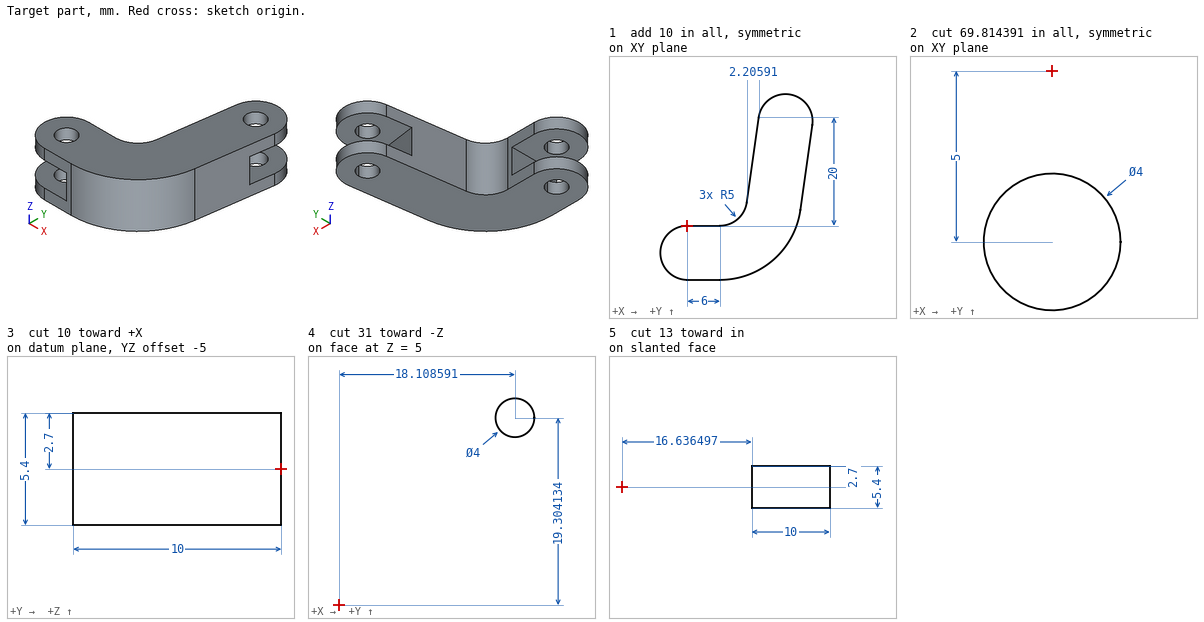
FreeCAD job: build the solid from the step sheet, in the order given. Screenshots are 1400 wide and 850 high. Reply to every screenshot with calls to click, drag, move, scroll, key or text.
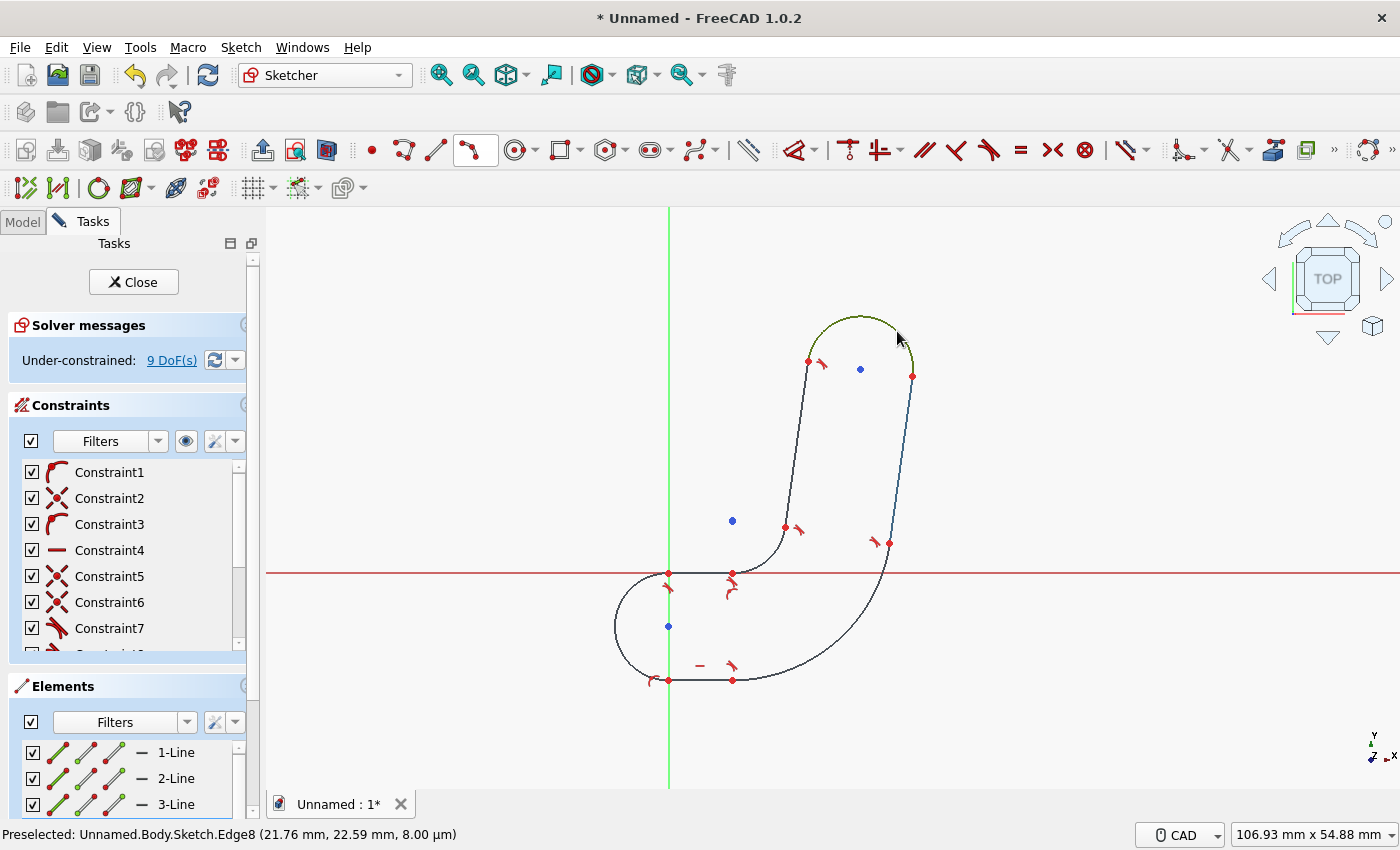
click(990, 150)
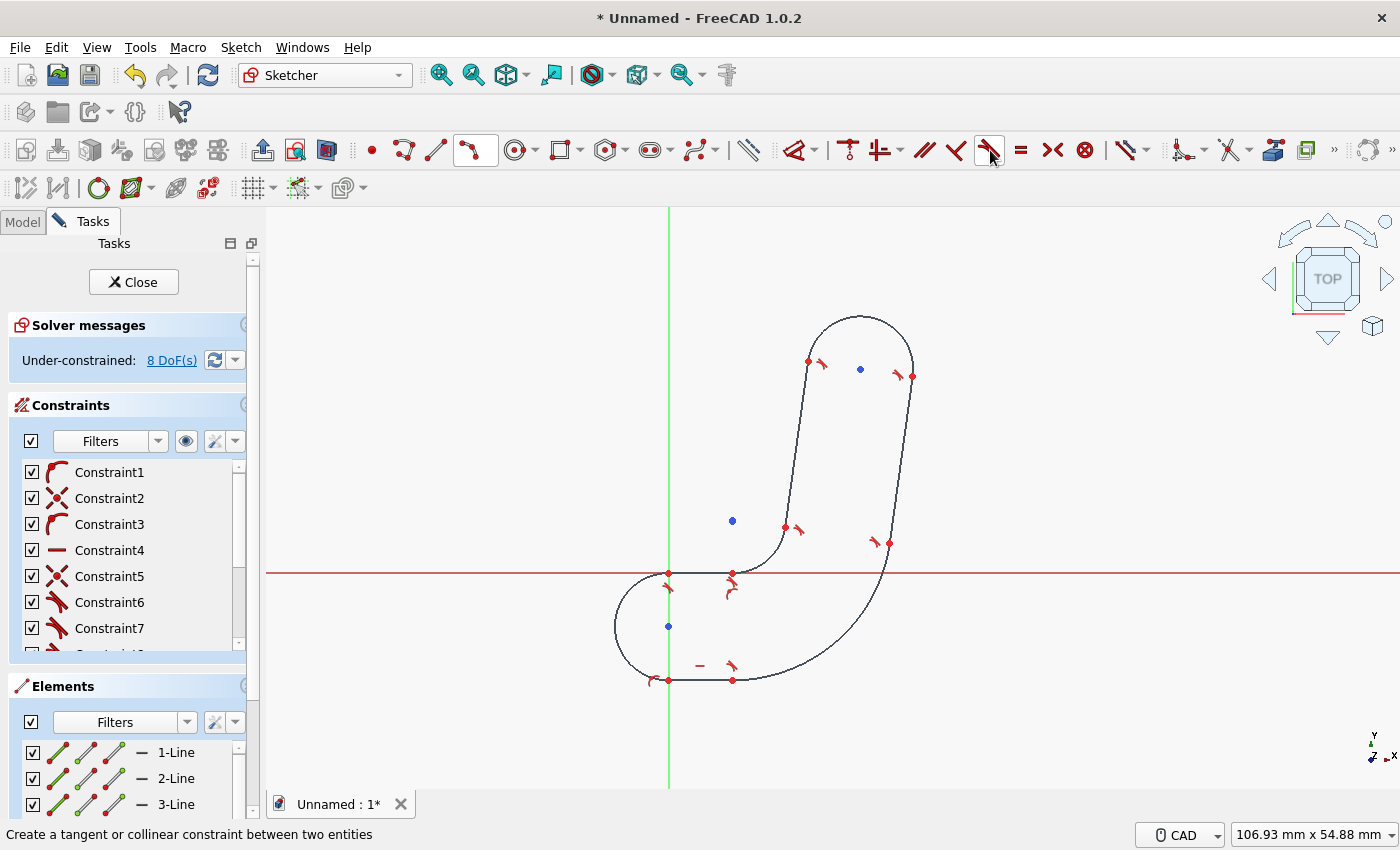
click(777, 549)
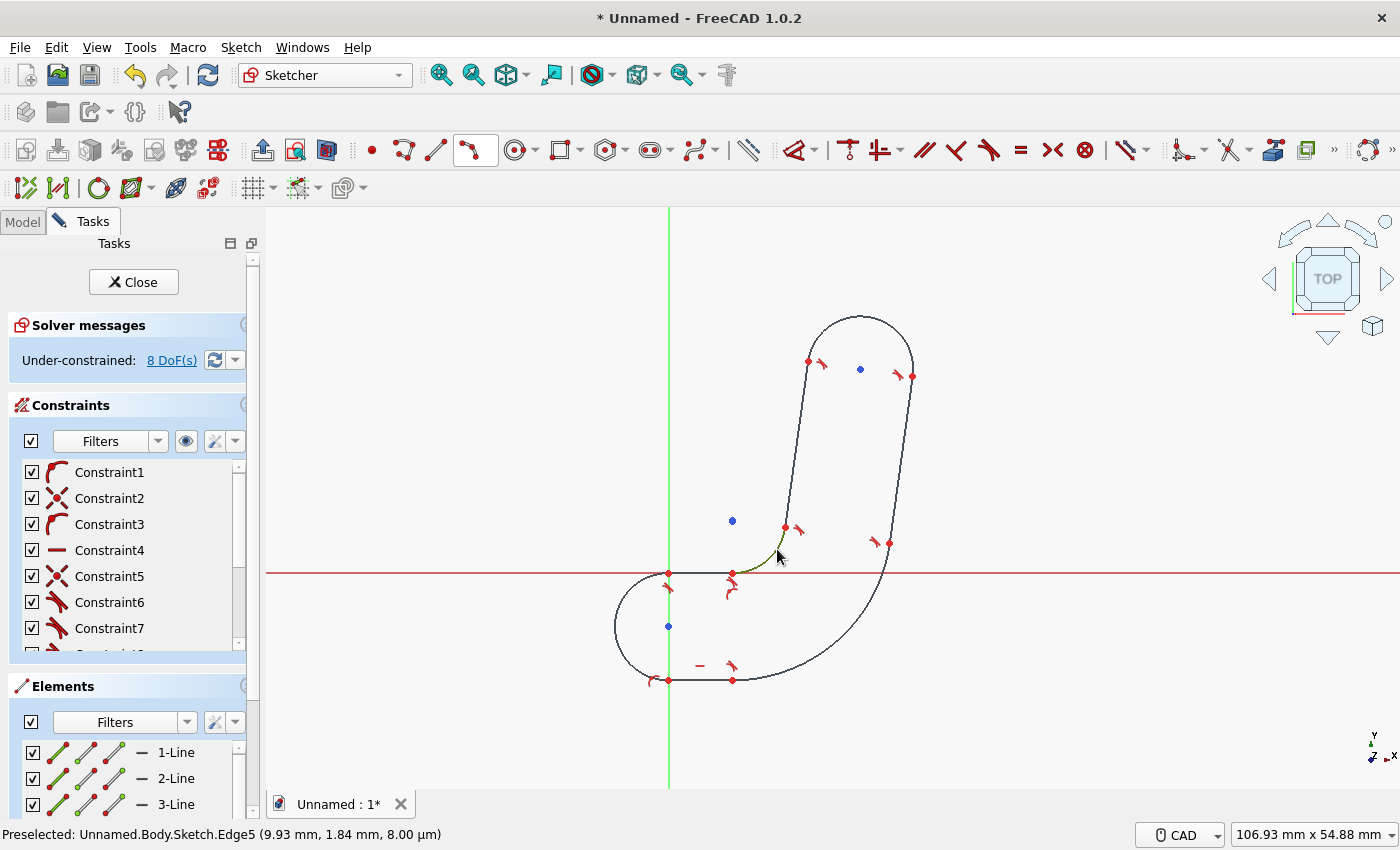
click(799, 666)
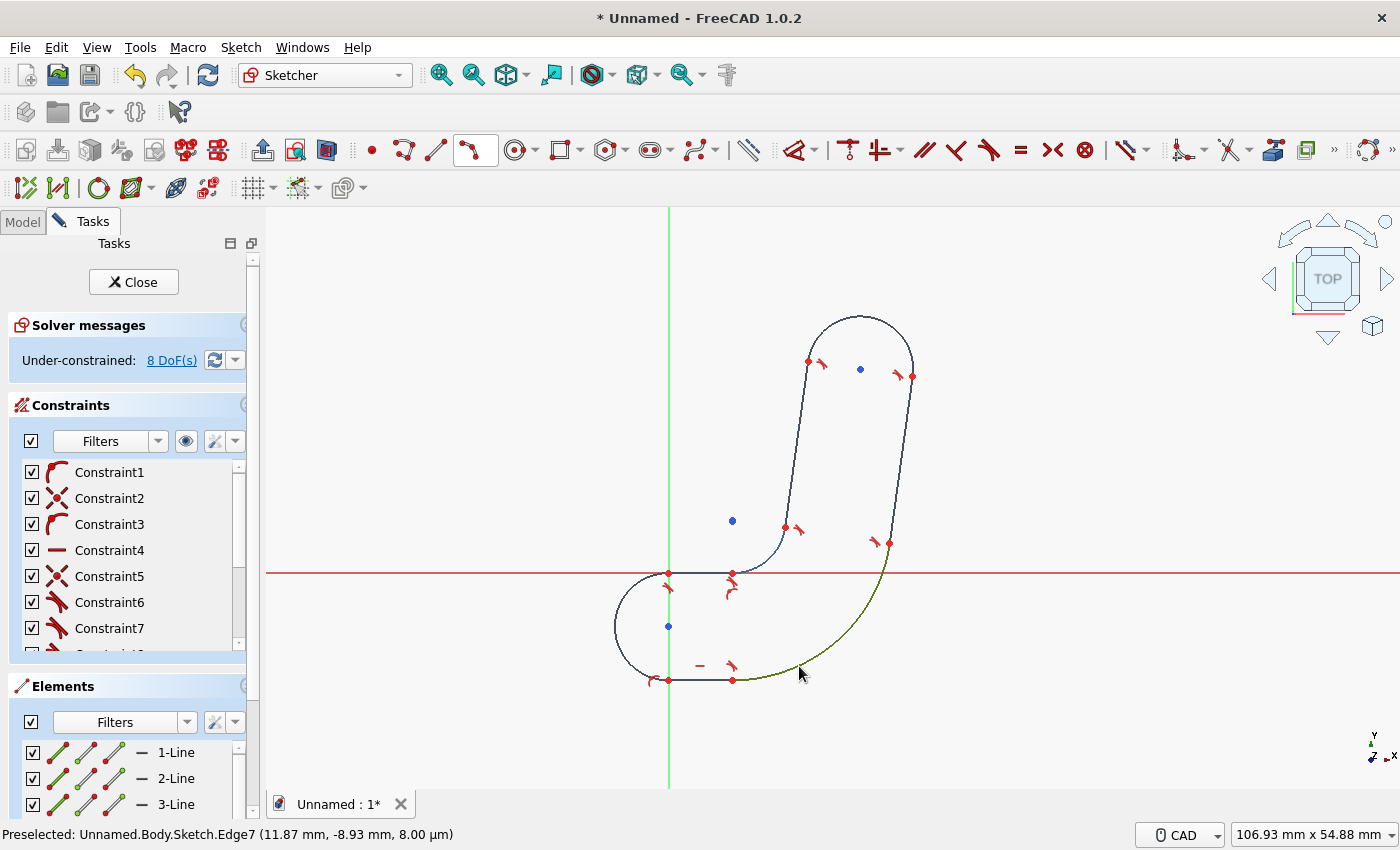
key(c)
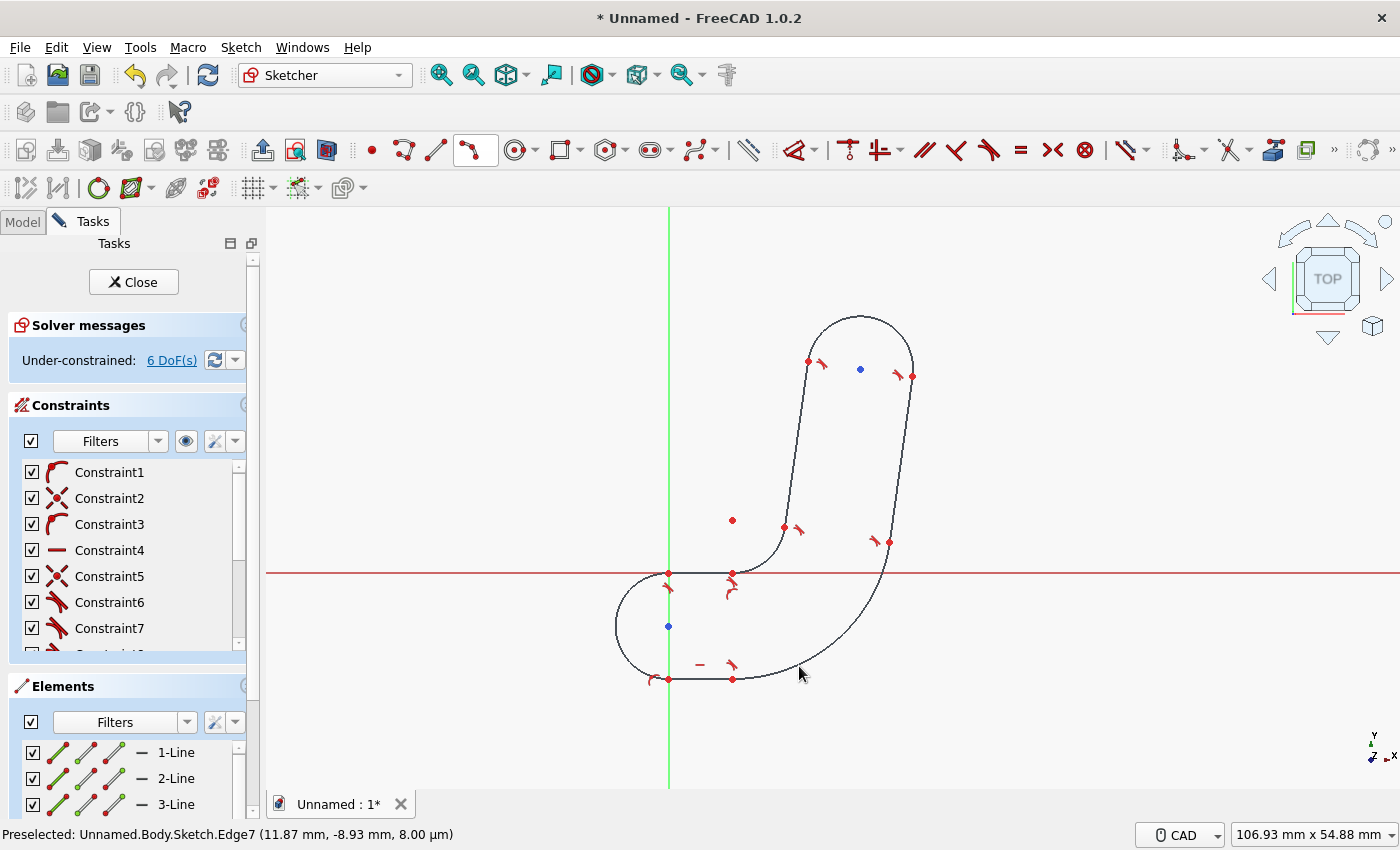
click(777, 549)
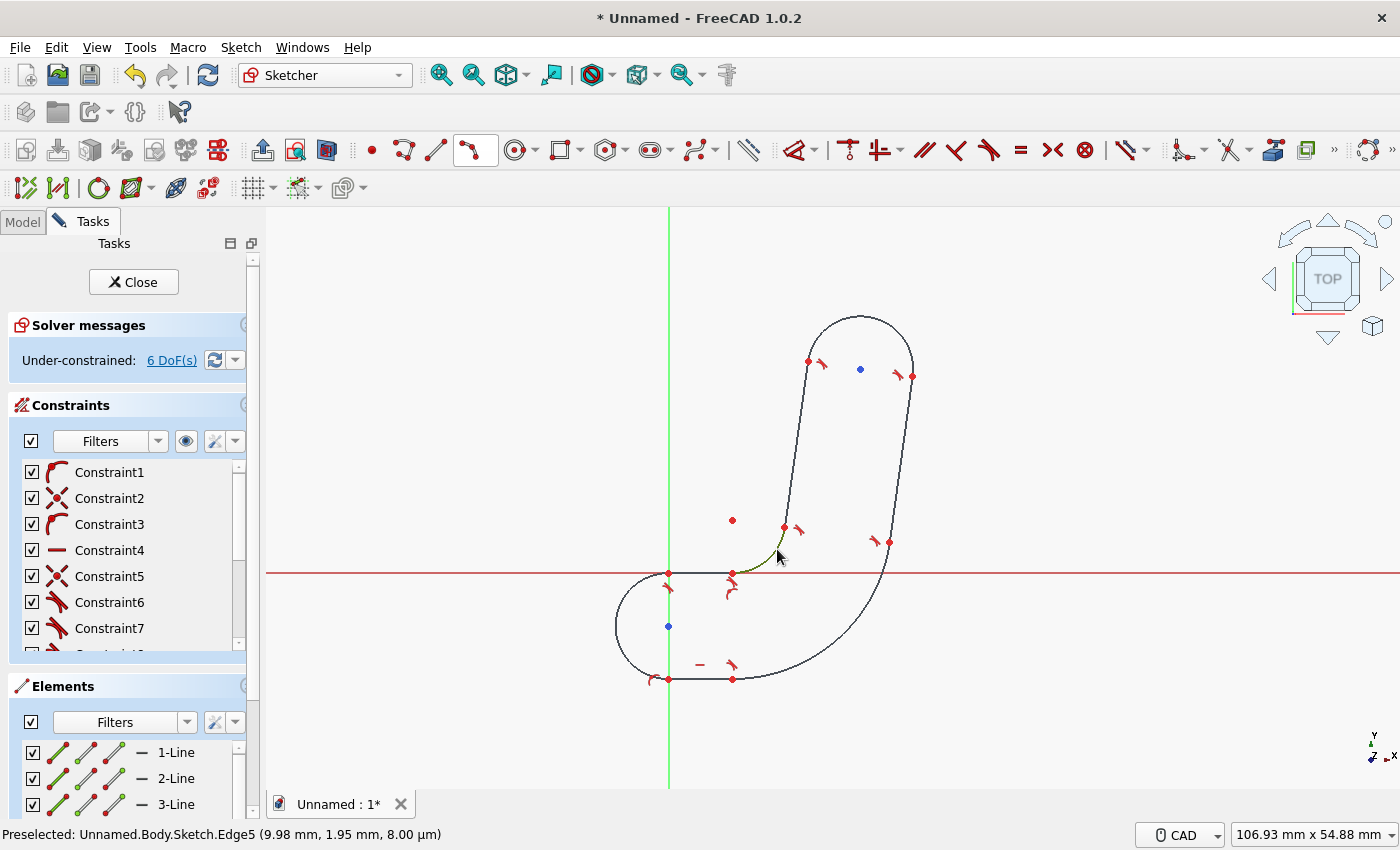
click(626, 595)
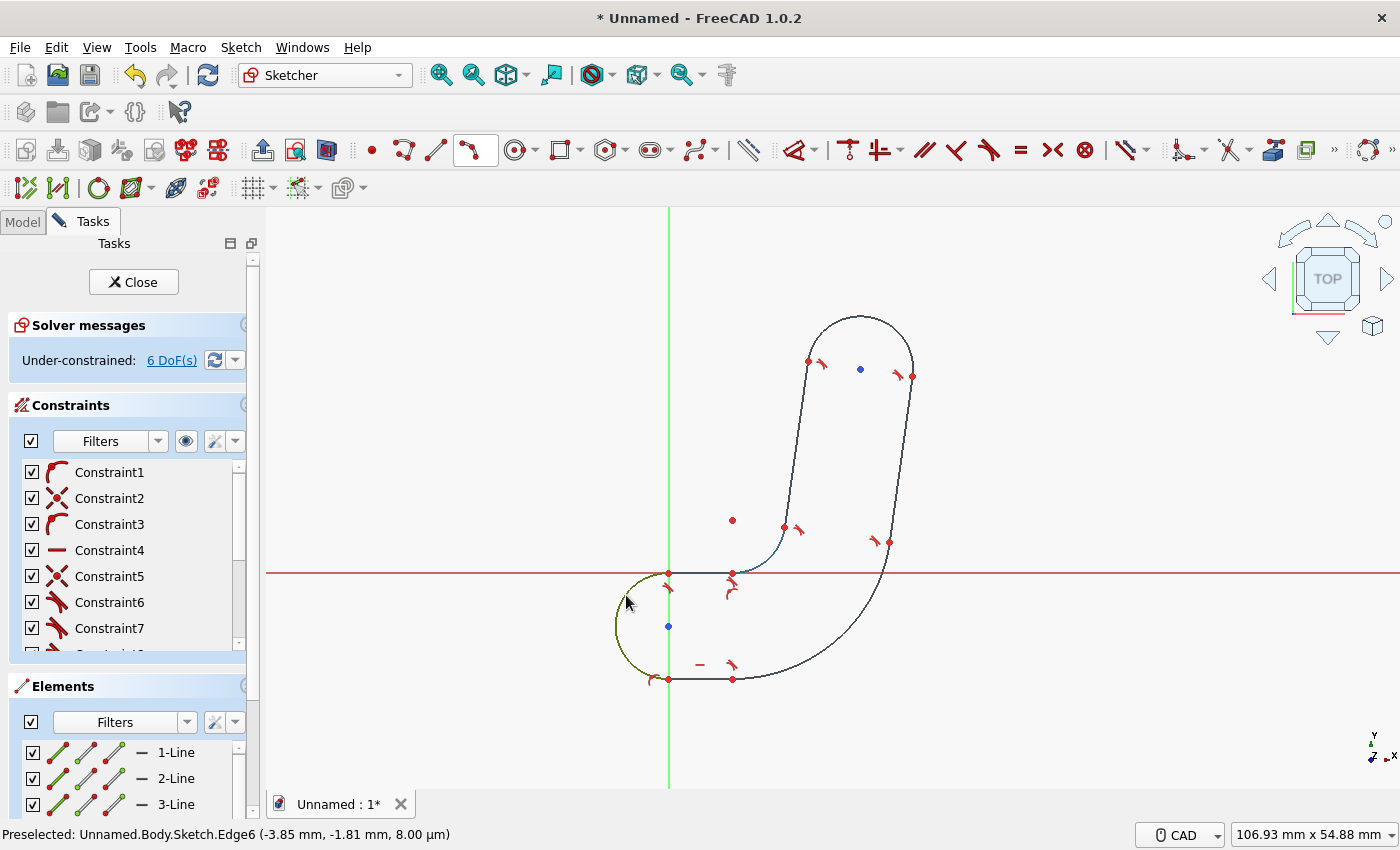
click(897, 331)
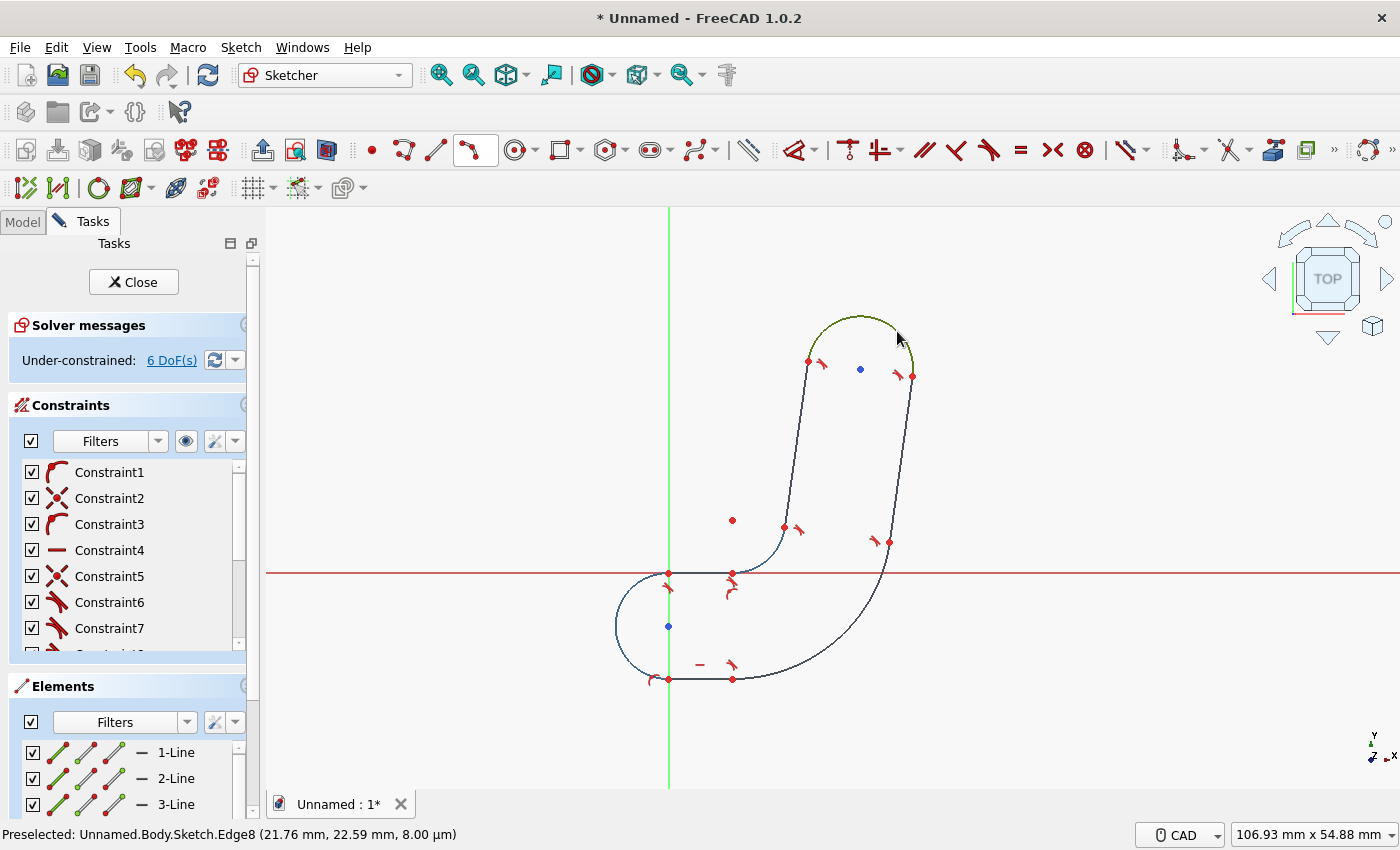
click(1022, 150)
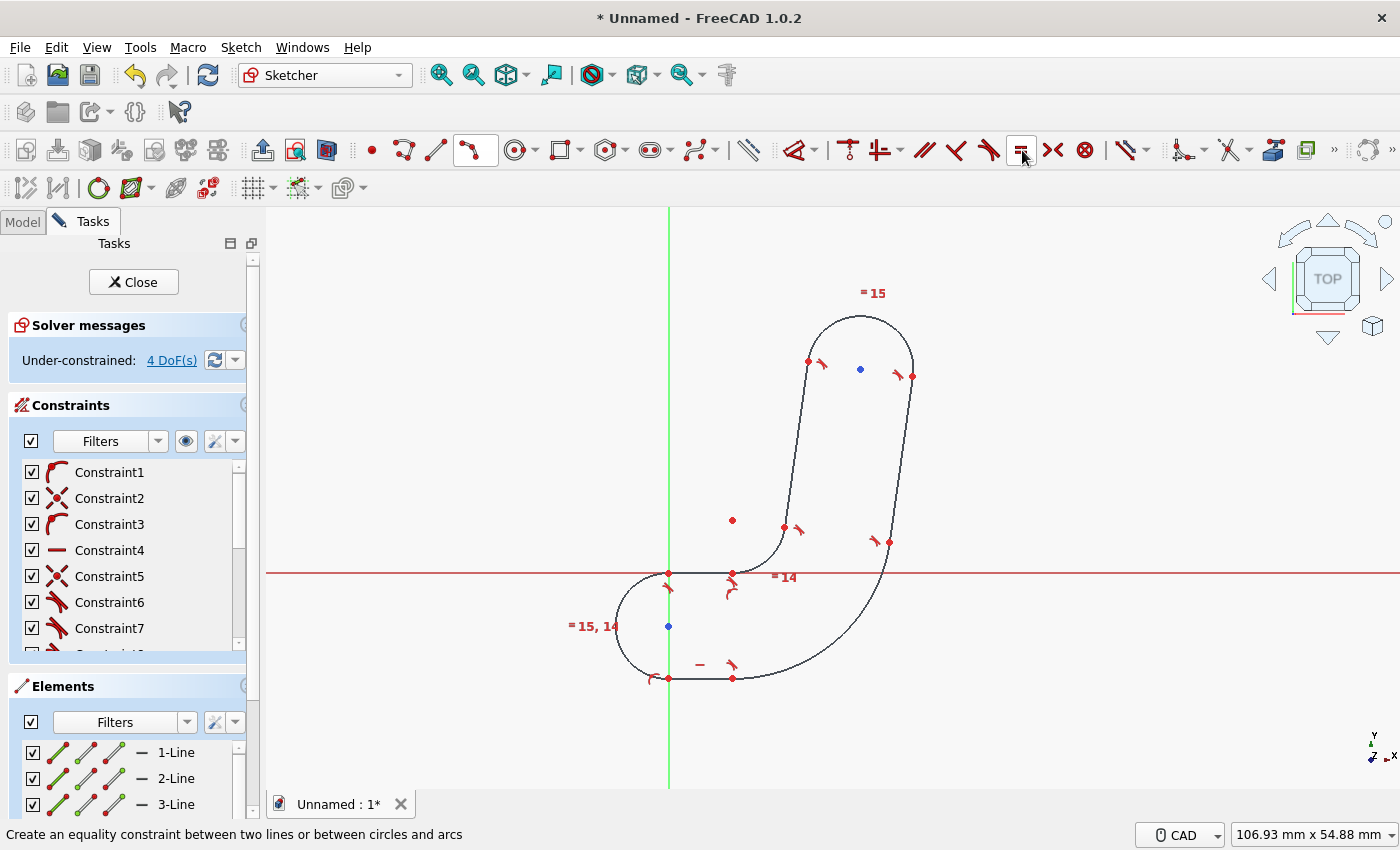
key(d)